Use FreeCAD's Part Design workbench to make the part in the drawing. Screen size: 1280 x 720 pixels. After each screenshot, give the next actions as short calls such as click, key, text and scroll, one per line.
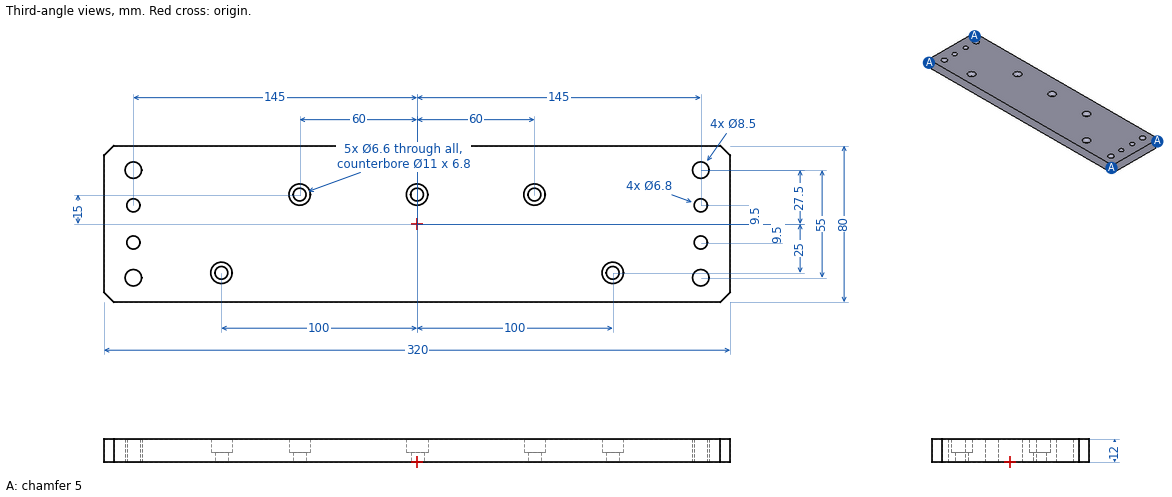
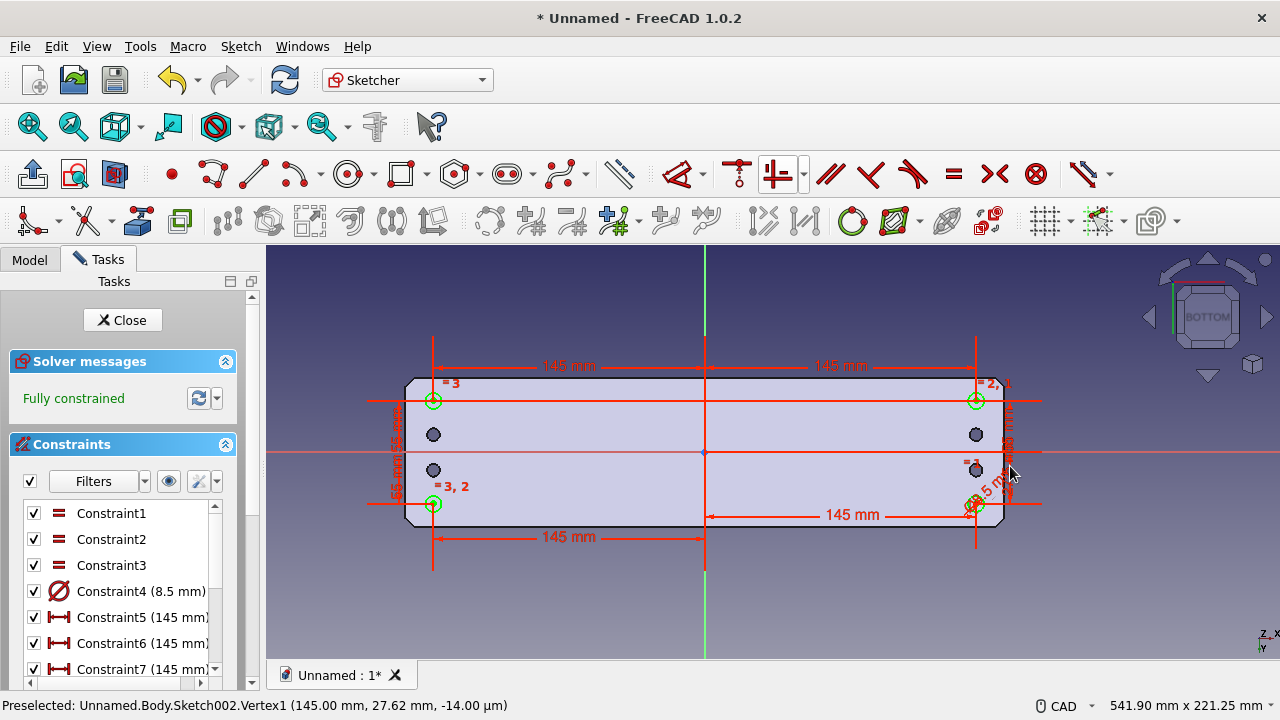
click(123, 320)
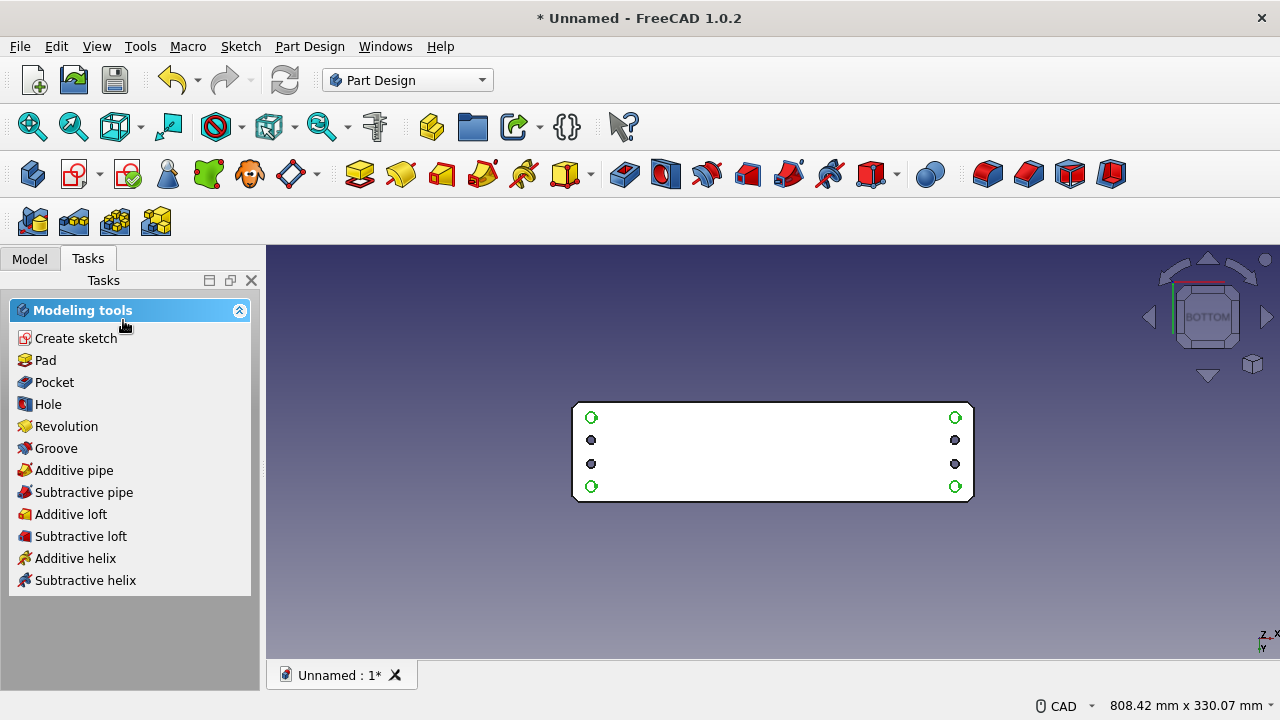
click(625, 174)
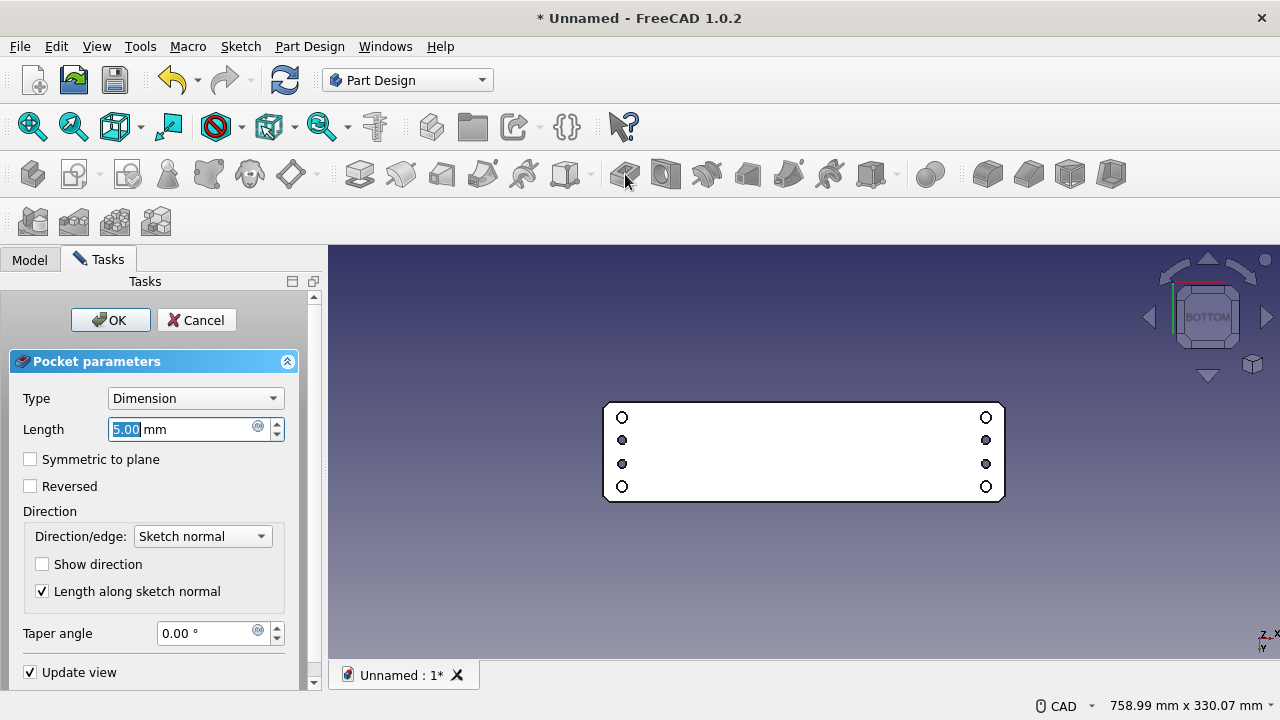
click(196, 398)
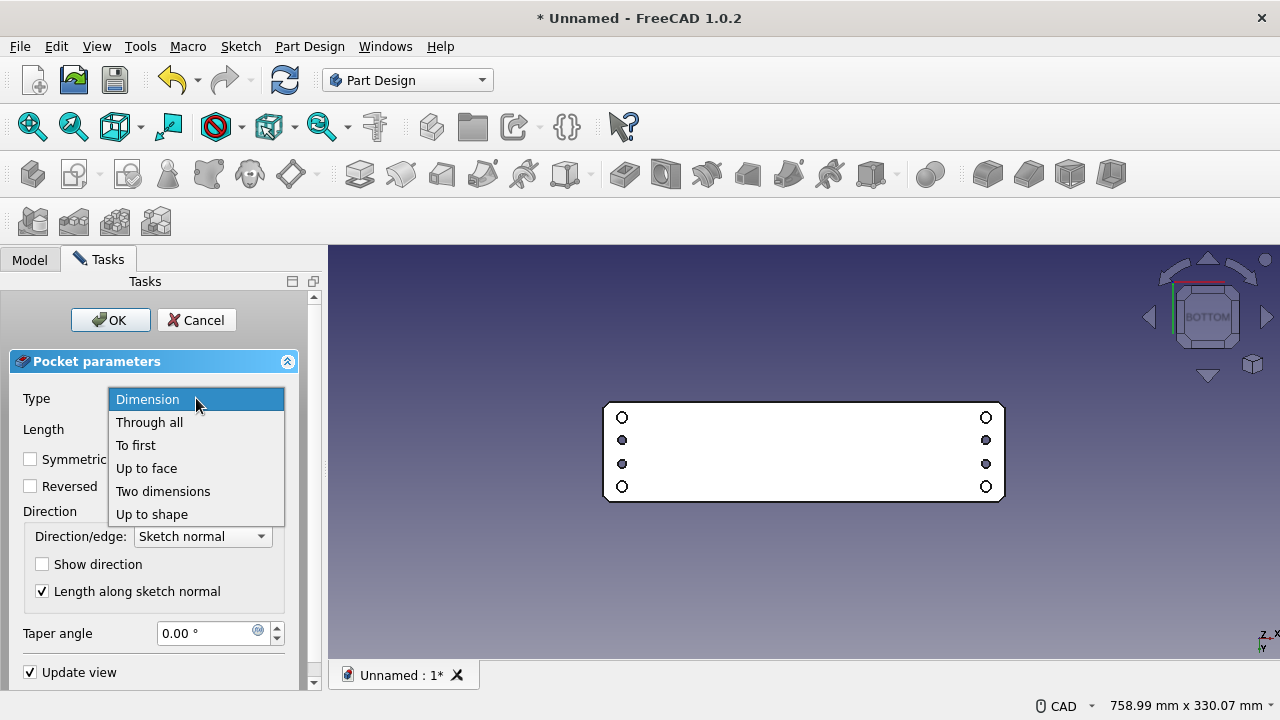
click(194, 422)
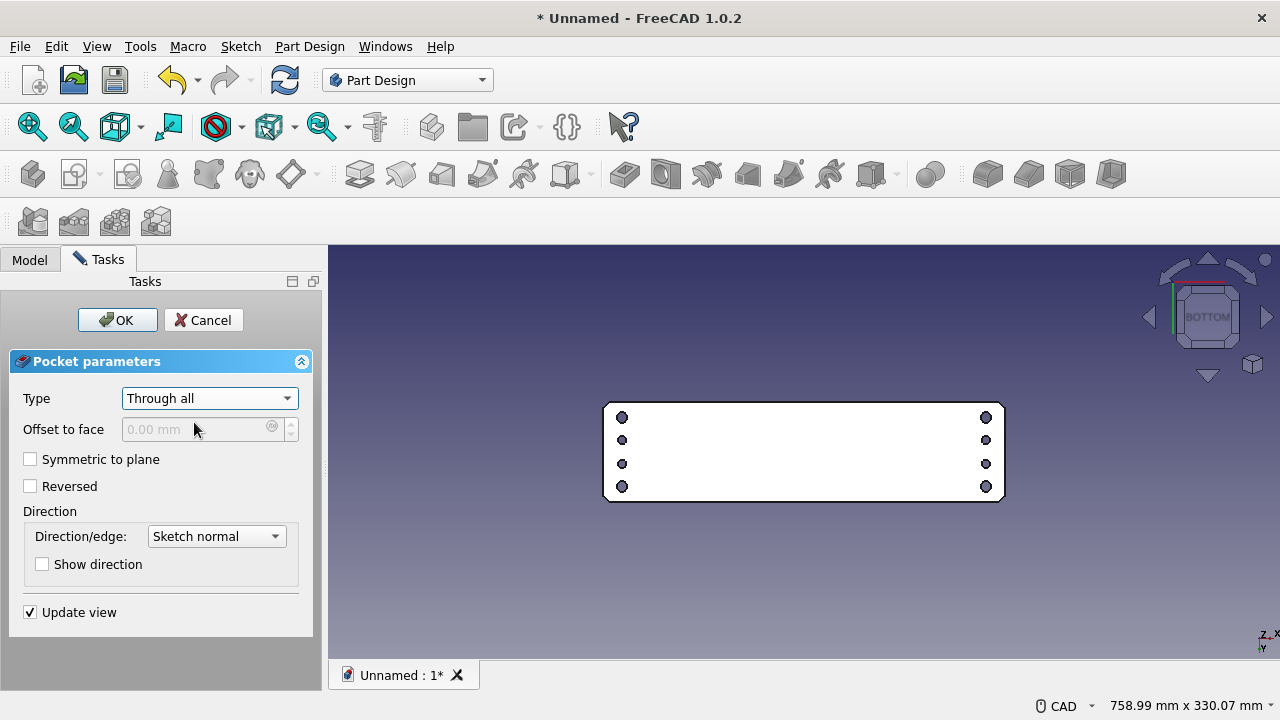
click(118, 320)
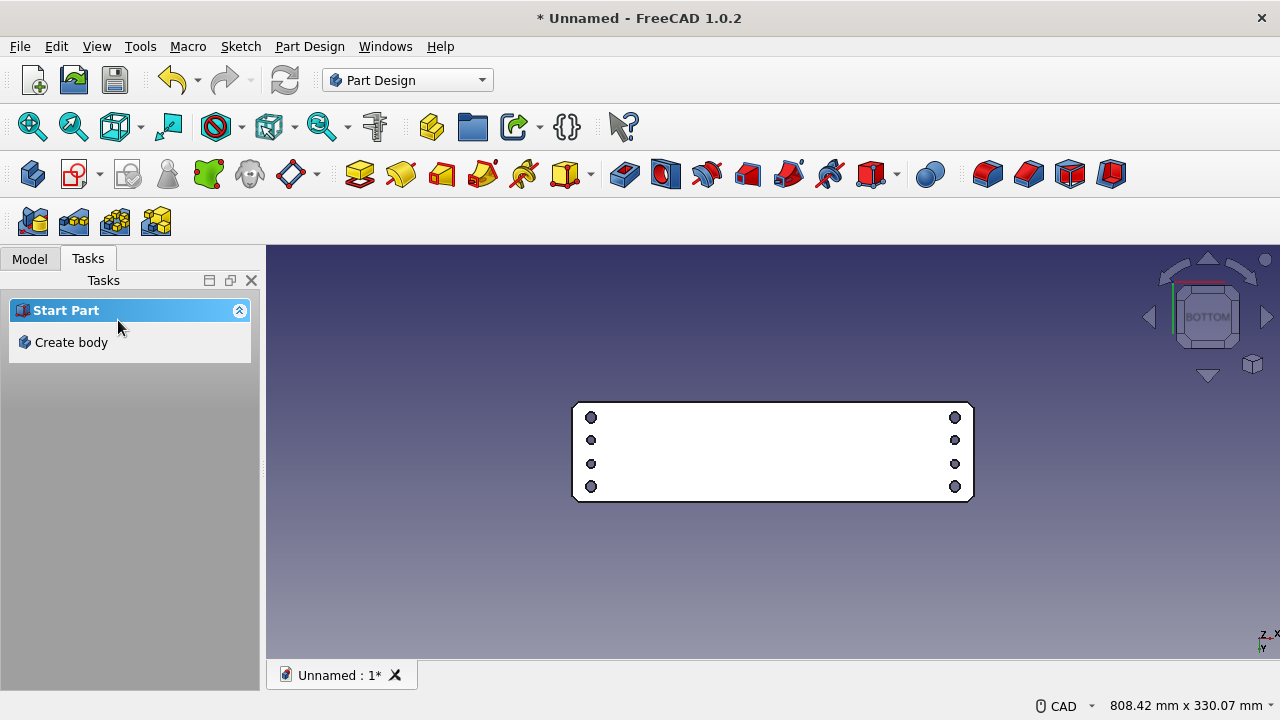
key(v)
key(f)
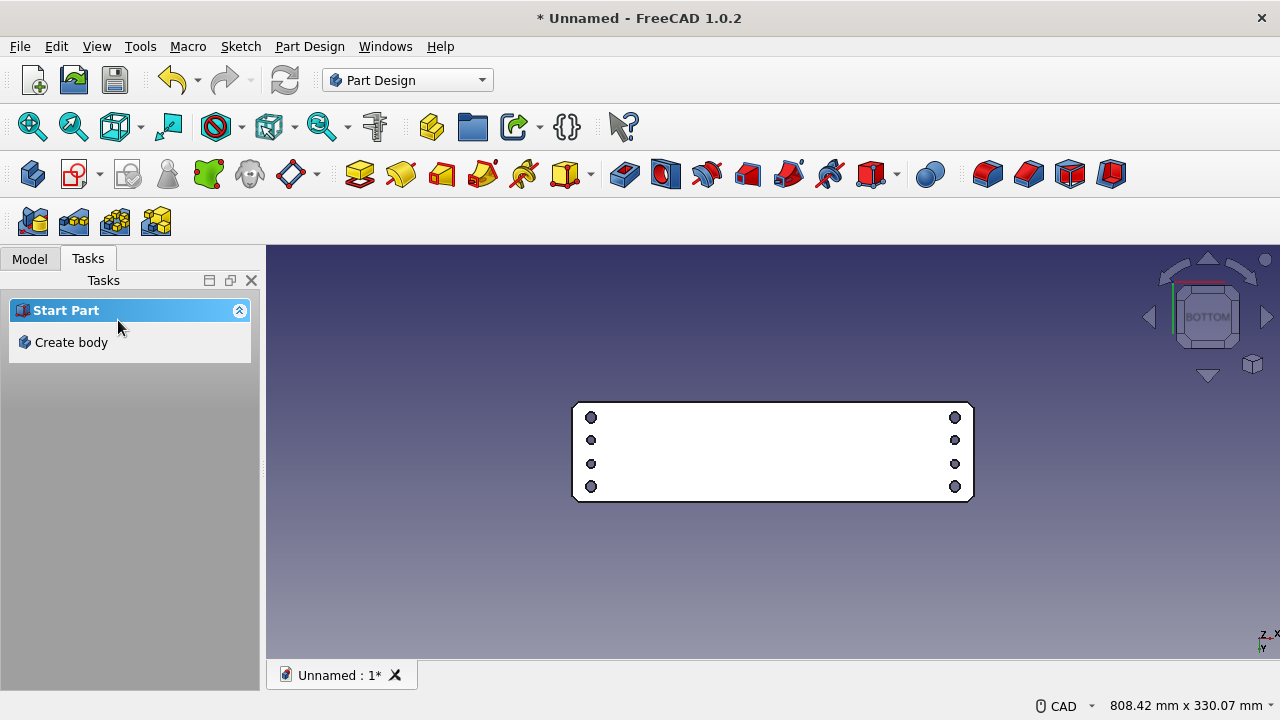
key(0)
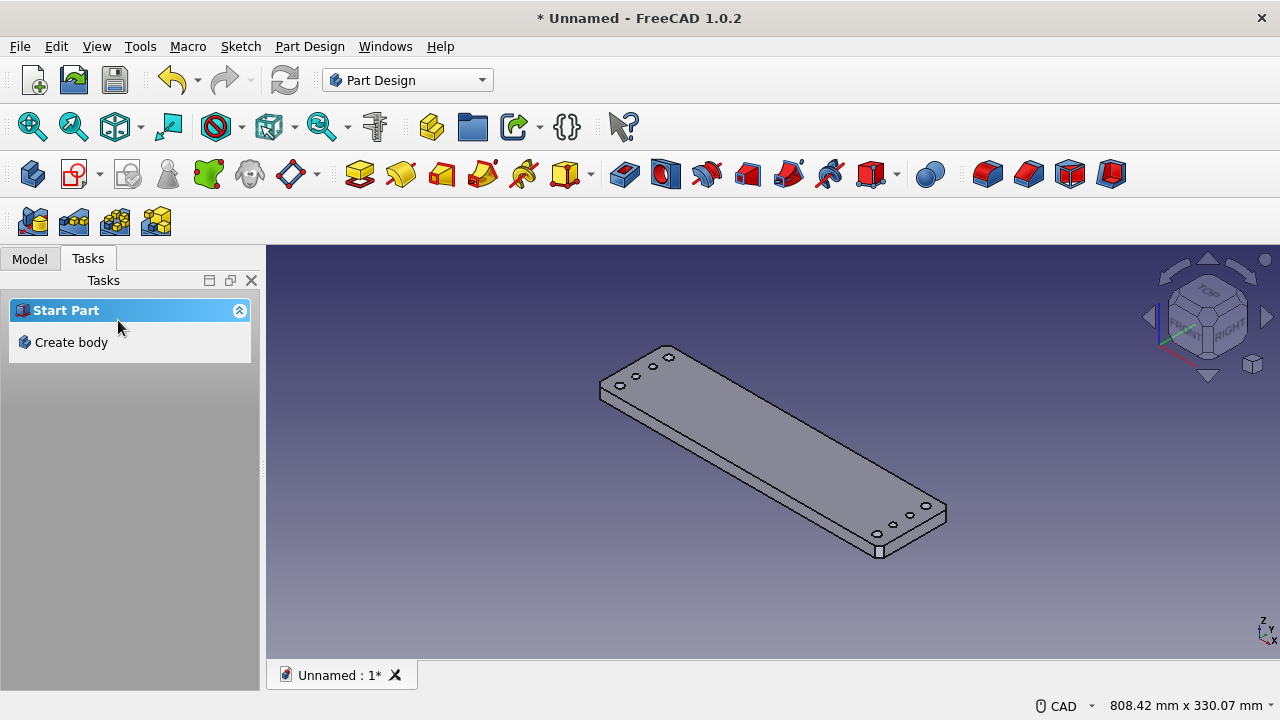
click(854, 492)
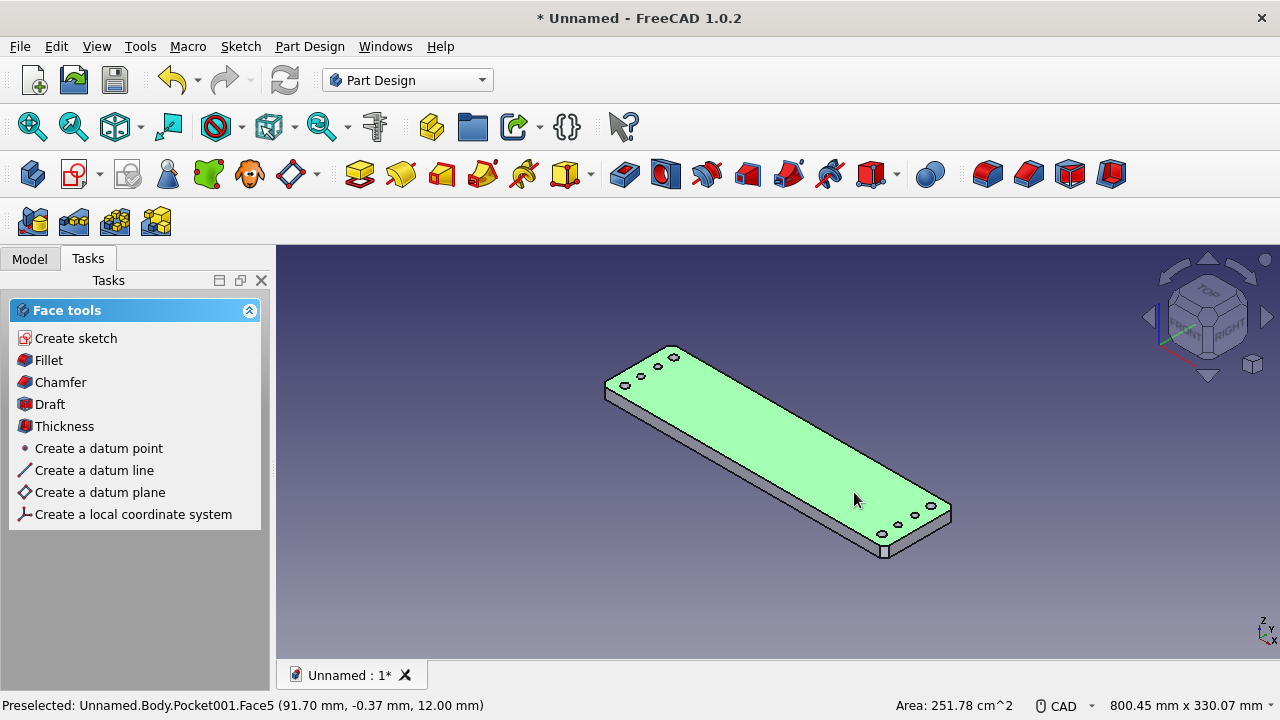
click(74, 174)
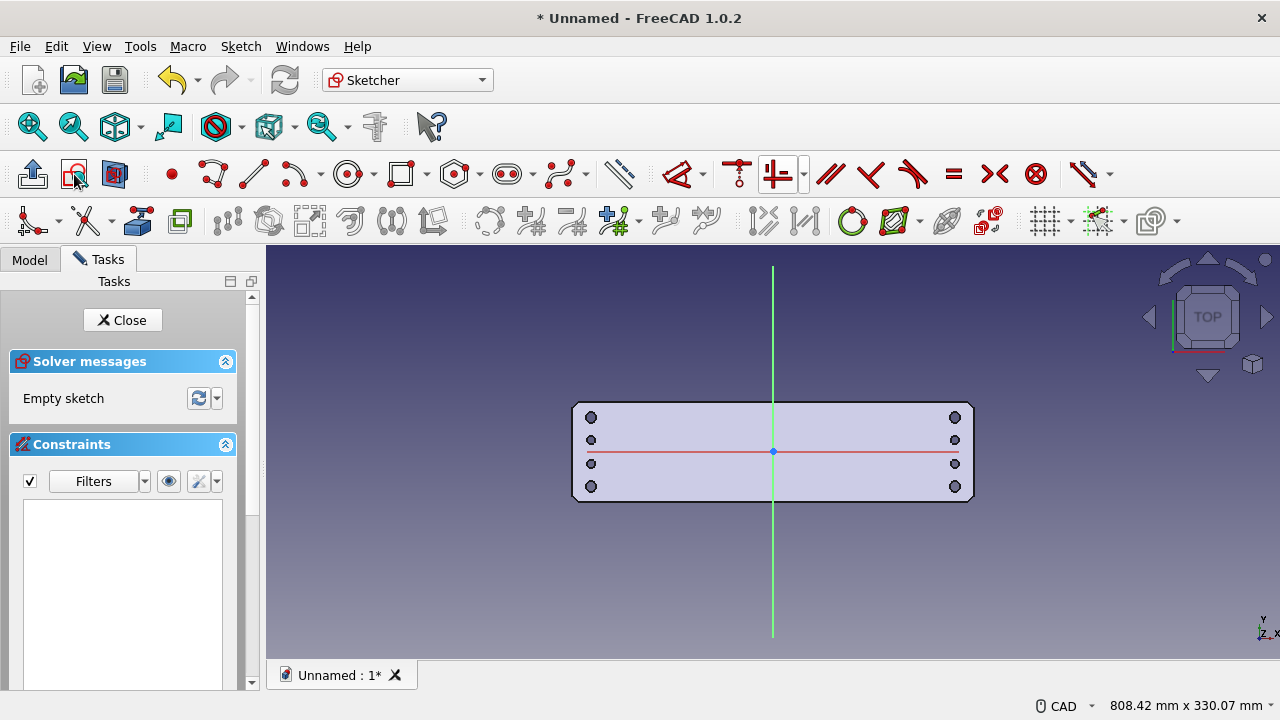
scroll(829, 463, up, 4)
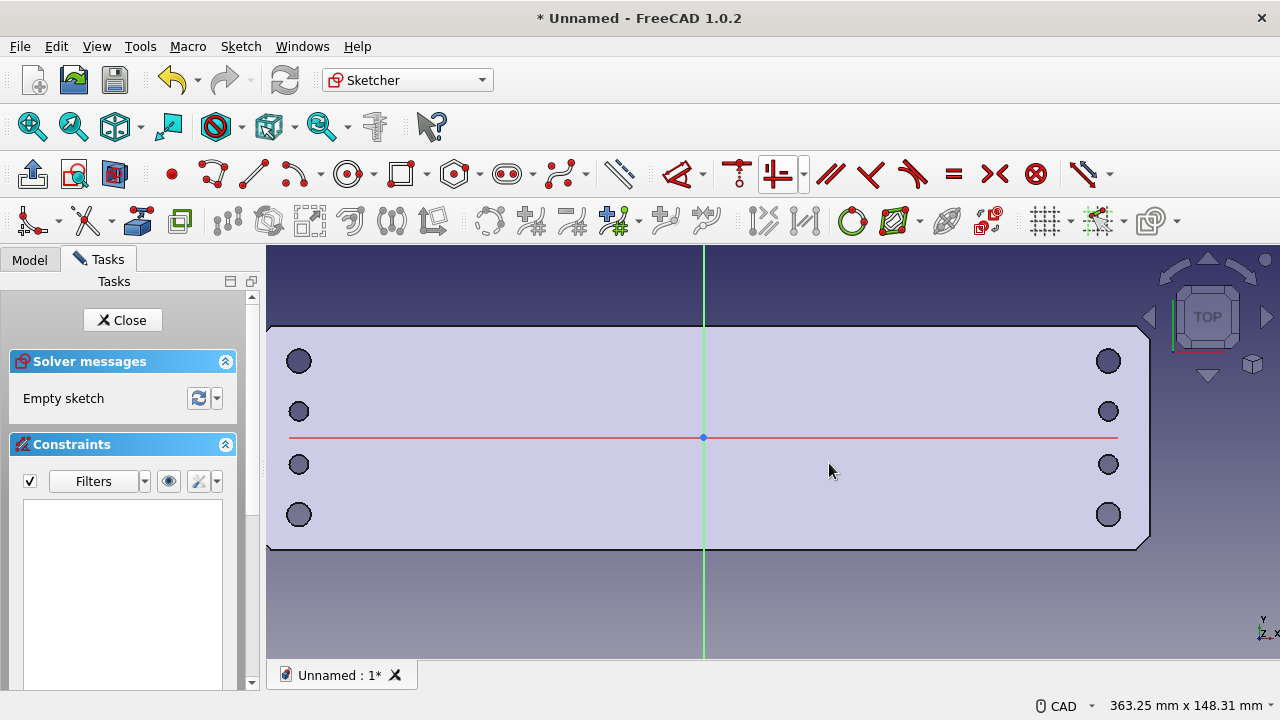
click(348, 174)